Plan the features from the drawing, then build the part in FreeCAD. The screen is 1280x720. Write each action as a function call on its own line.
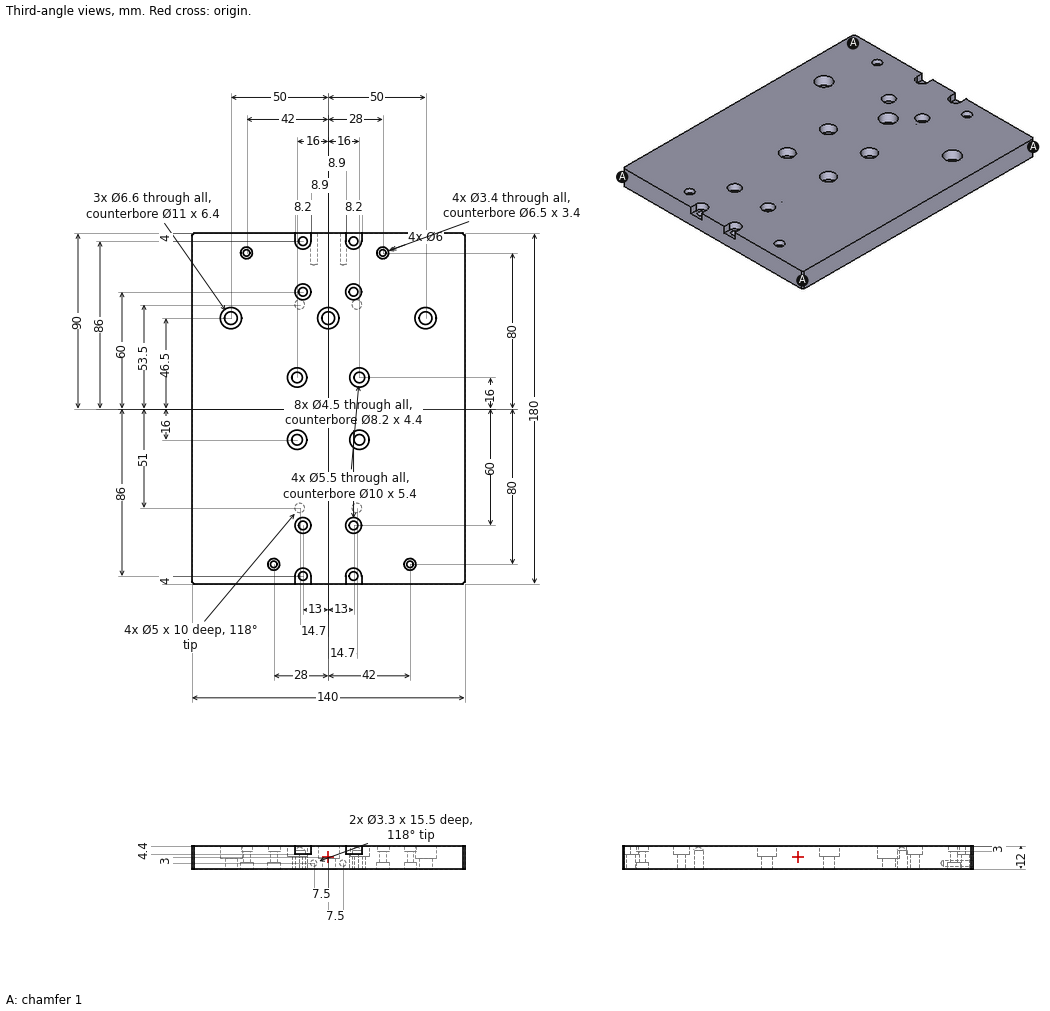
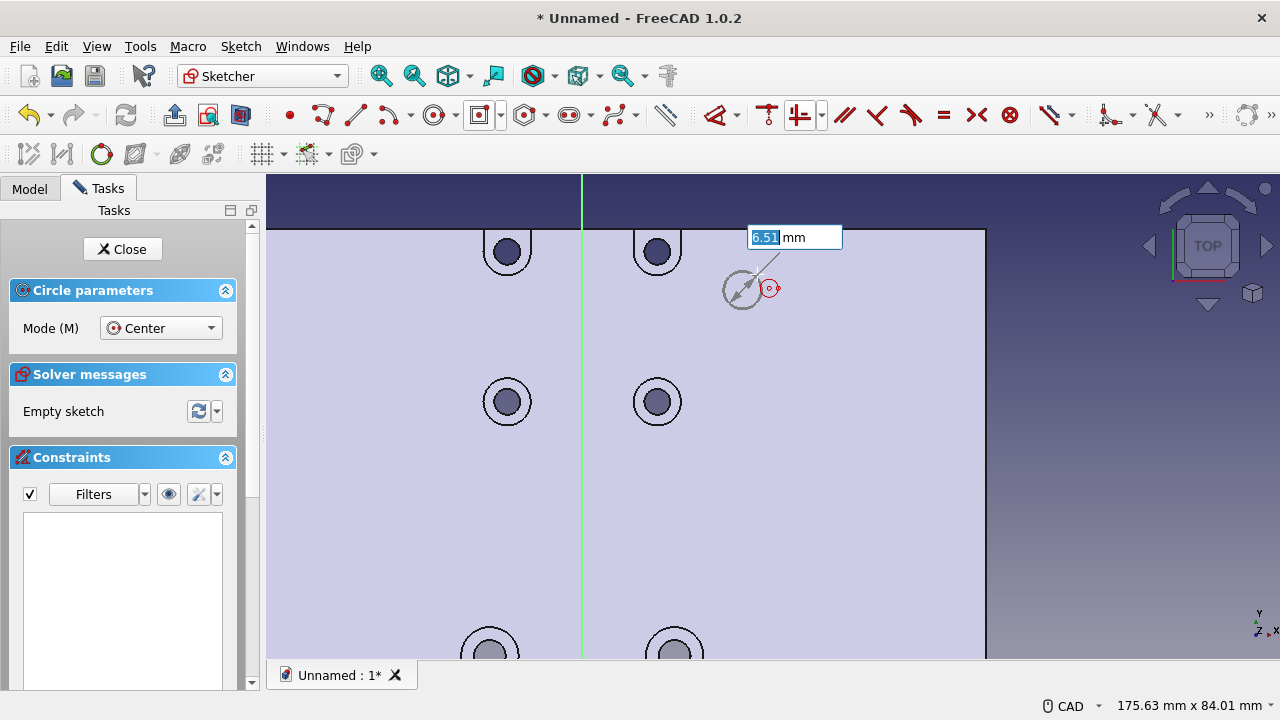
click(756, 274)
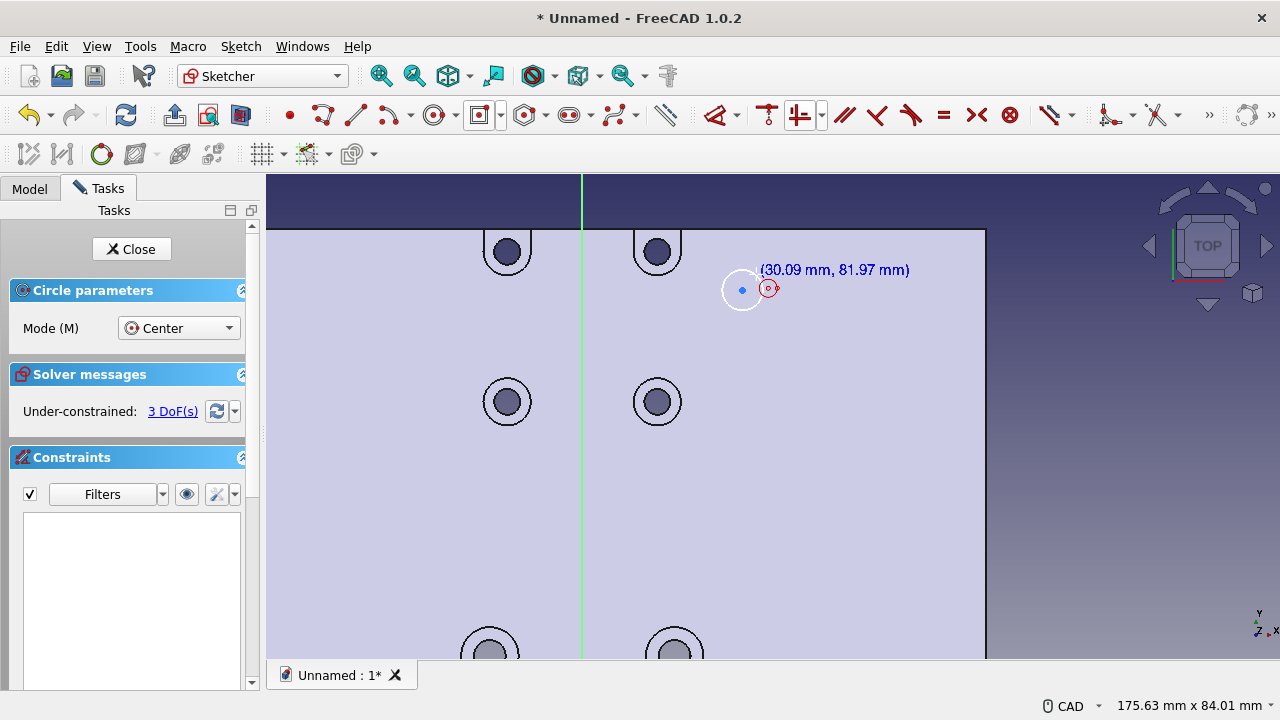
scroll(340, 286, up, 2)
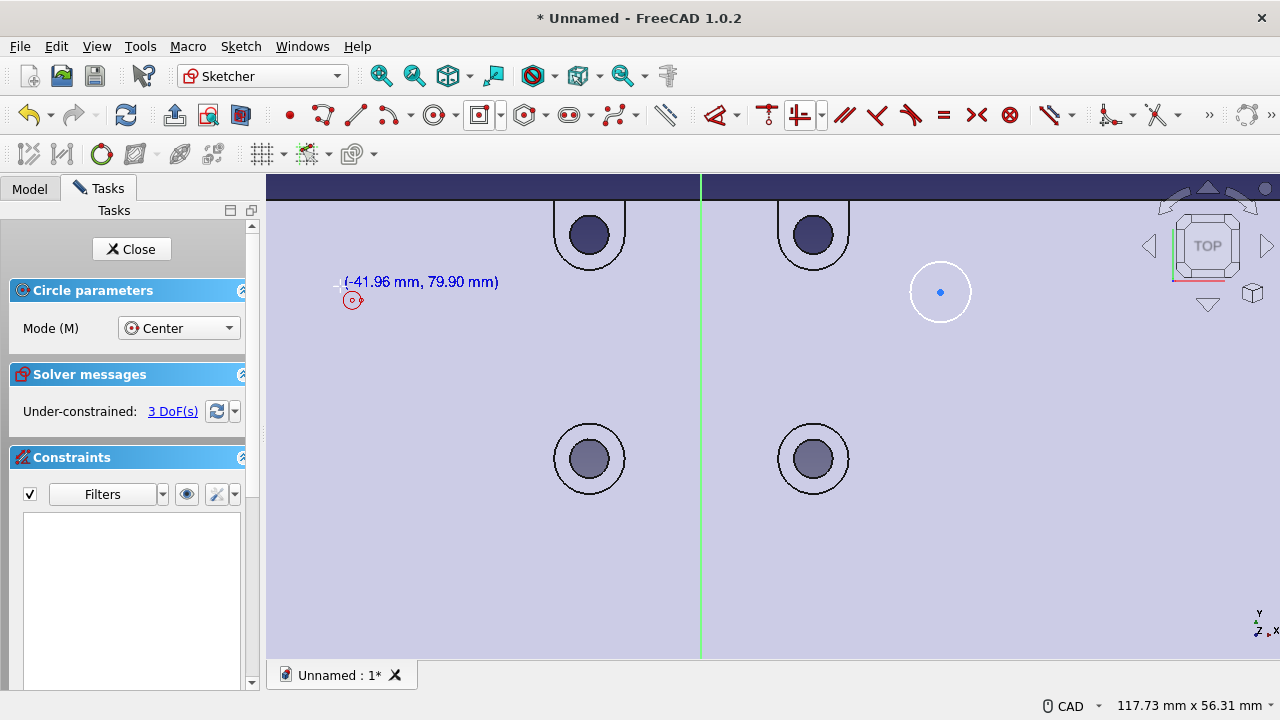
scroll(705, 275, down, 8)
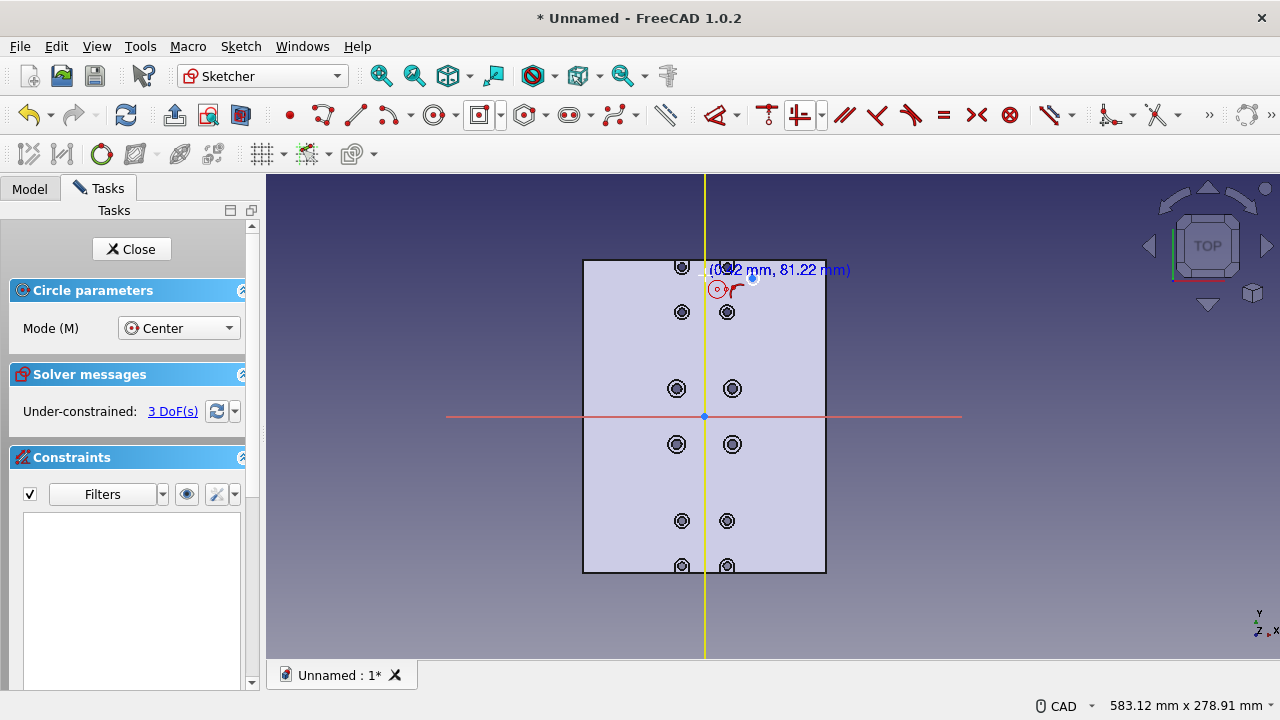
click(632, 277)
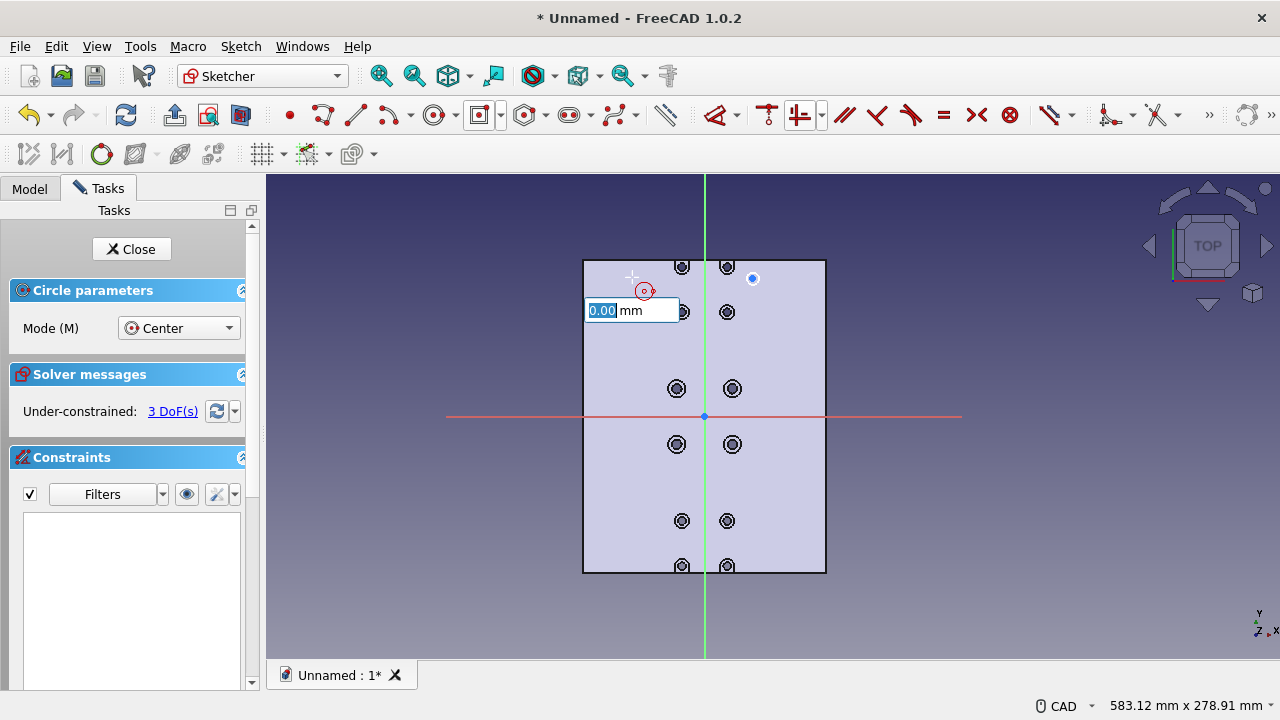
scroll(635, 274, up, 6)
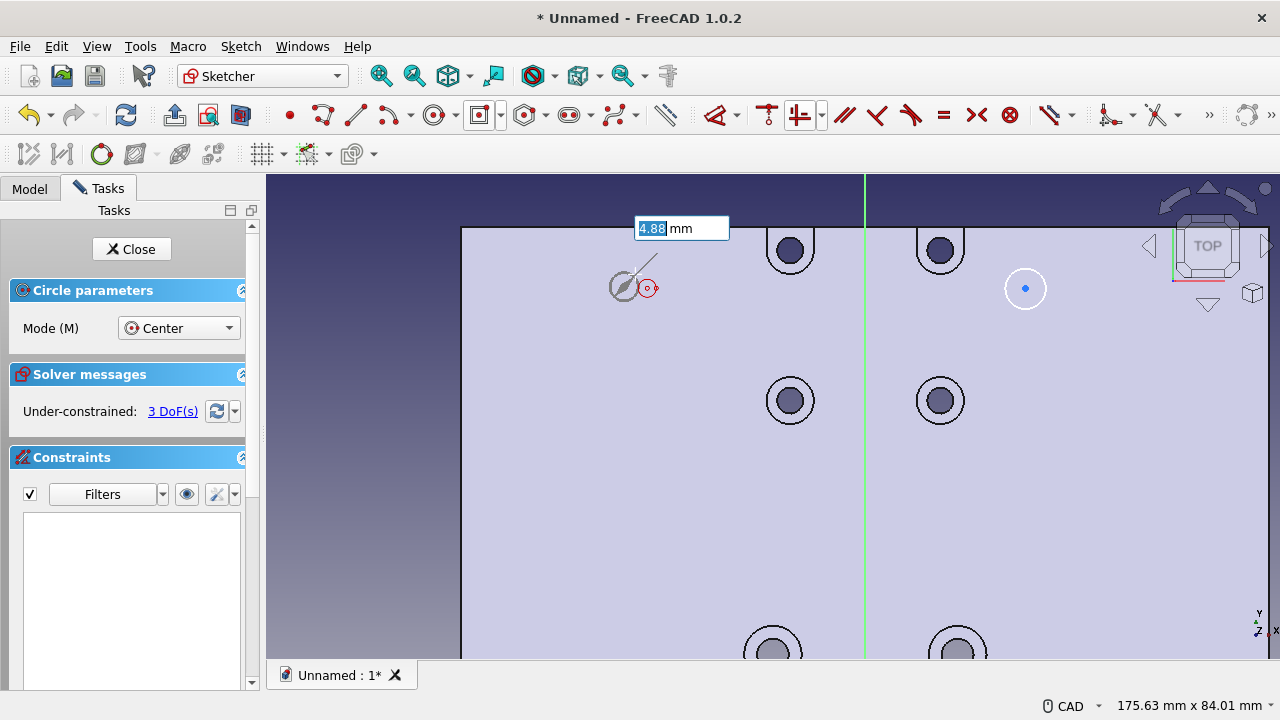
click(635, 273)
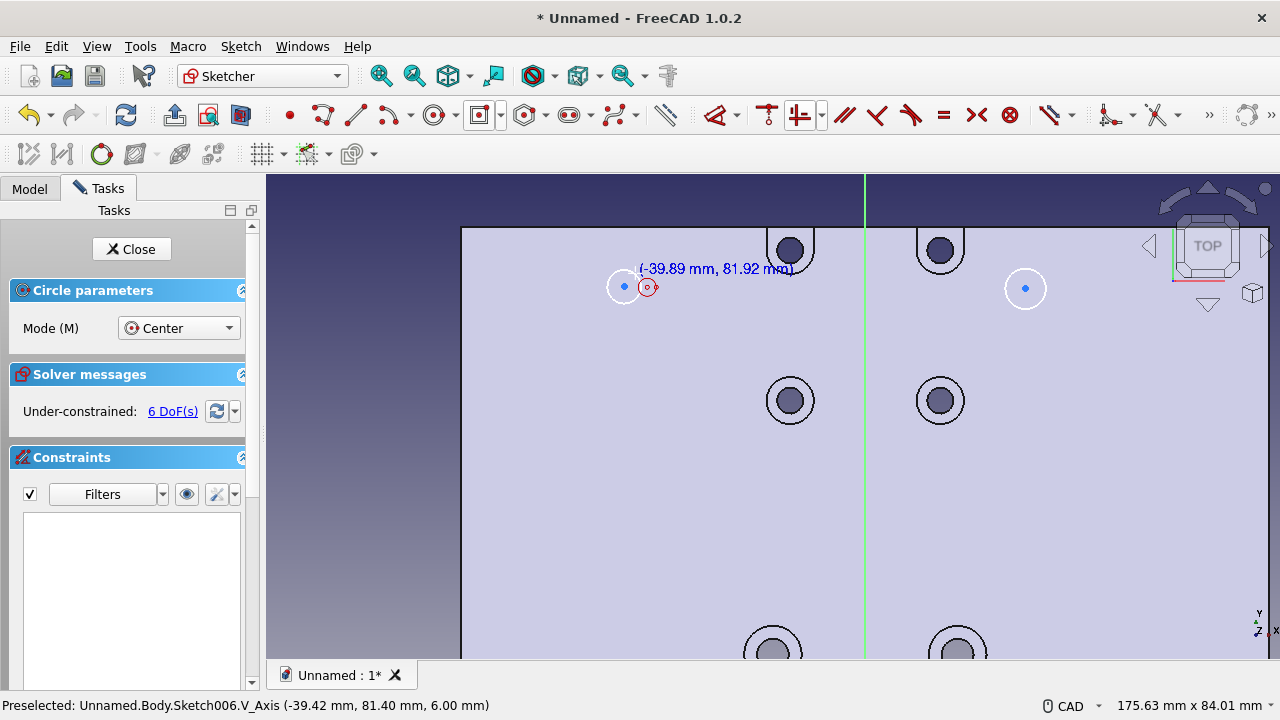
scroll(635, 274, down, 6)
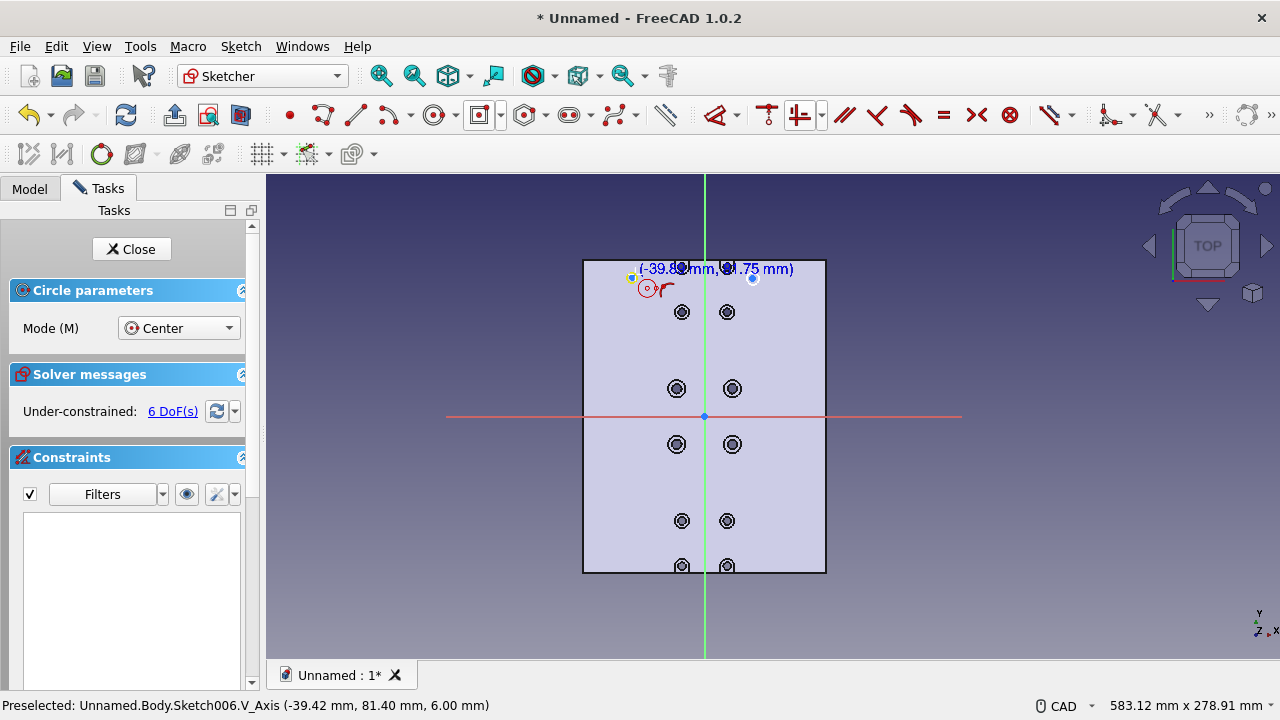
scroll(778, 556, up, 8)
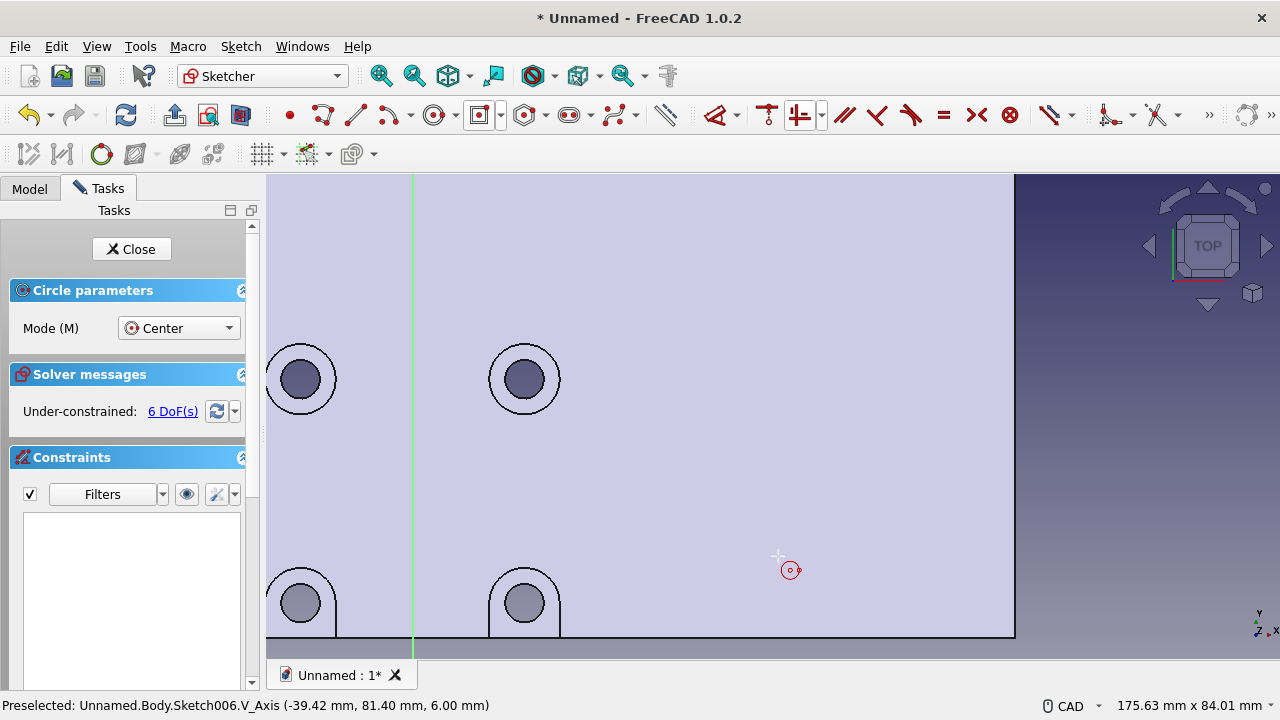
scroll(778, 557, down, 8)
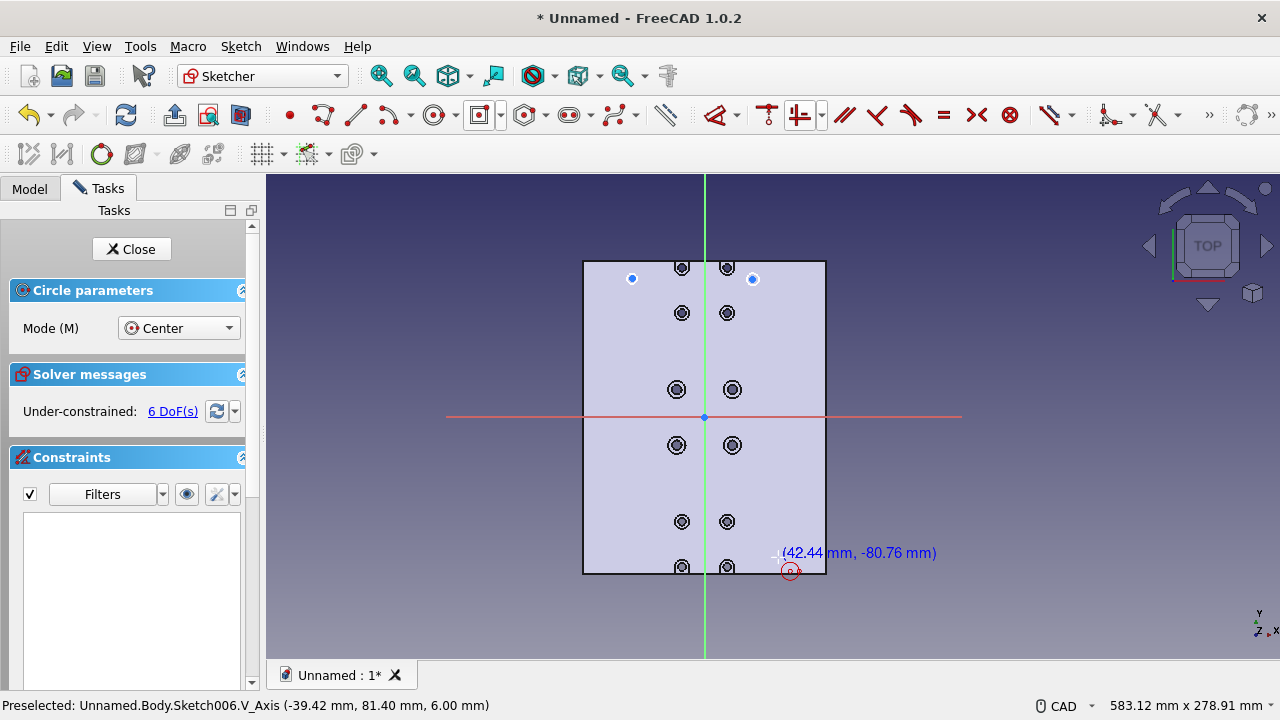
click(778, 557)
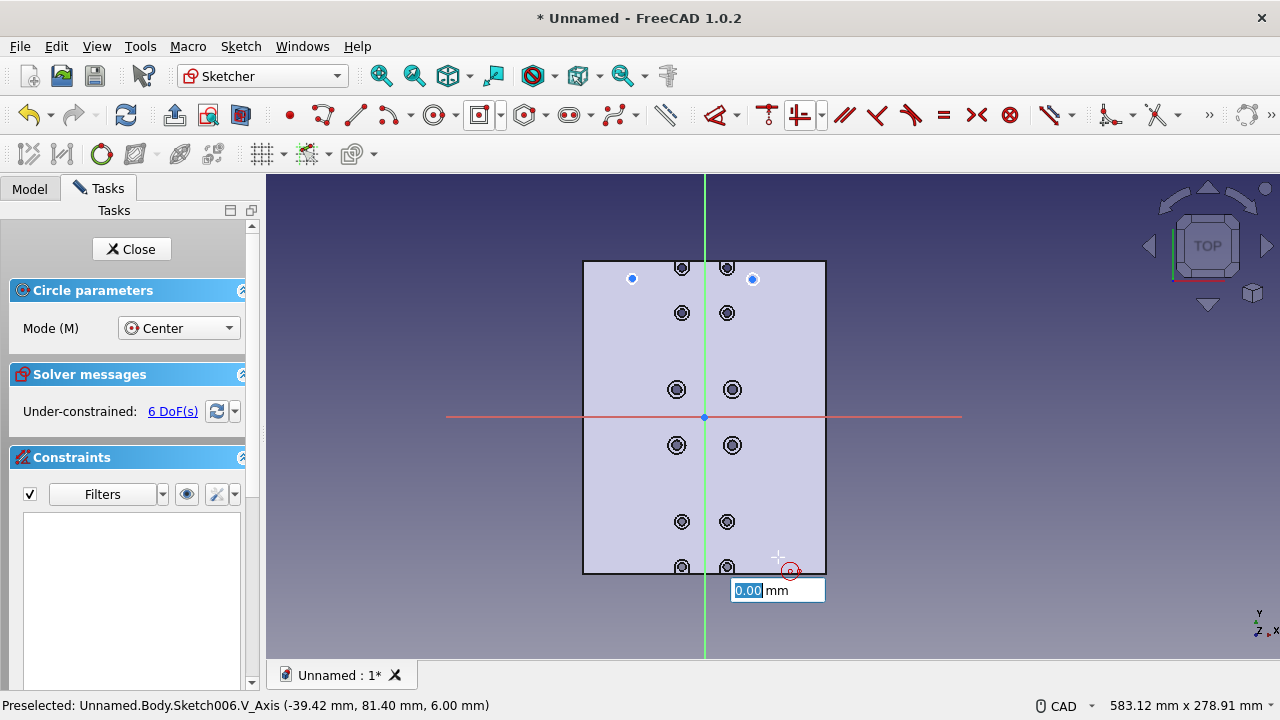
scroll(781, 553, up, 6)